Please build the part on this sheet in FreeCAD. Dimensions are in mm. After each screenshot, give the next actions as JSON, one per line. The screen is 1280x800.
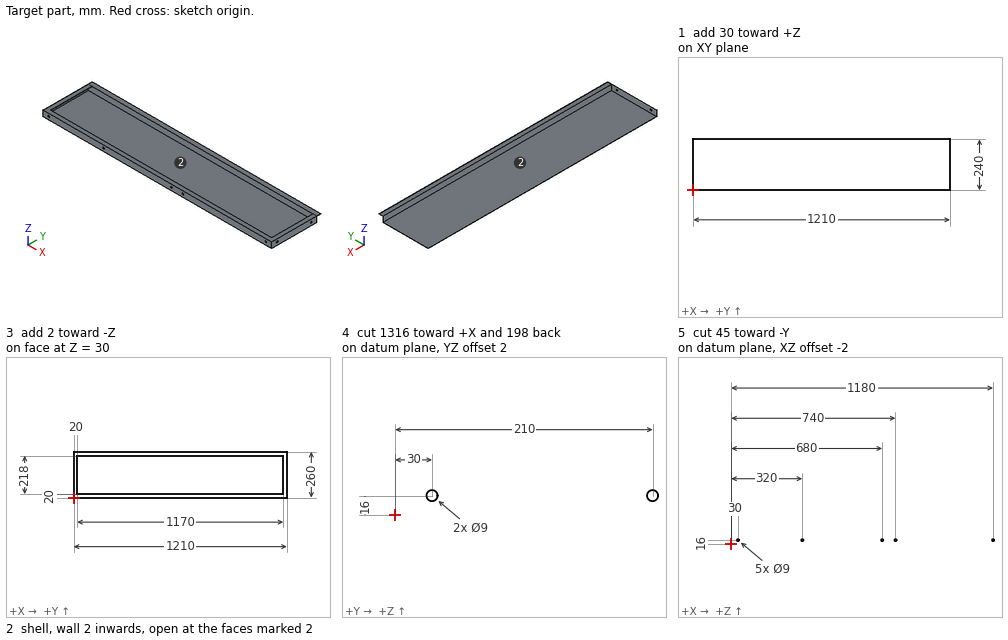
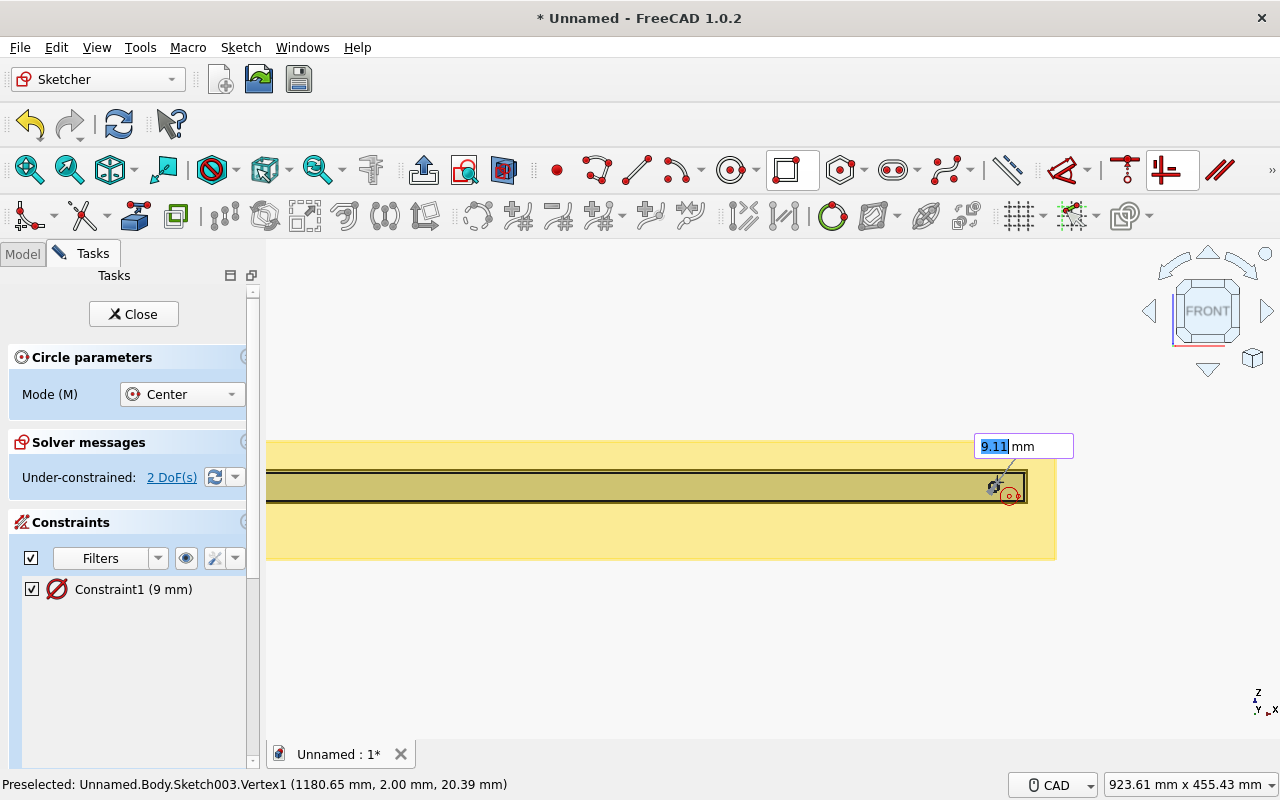
{"action": "type", "text": "9"}
{"action": "key", "text": "Return"}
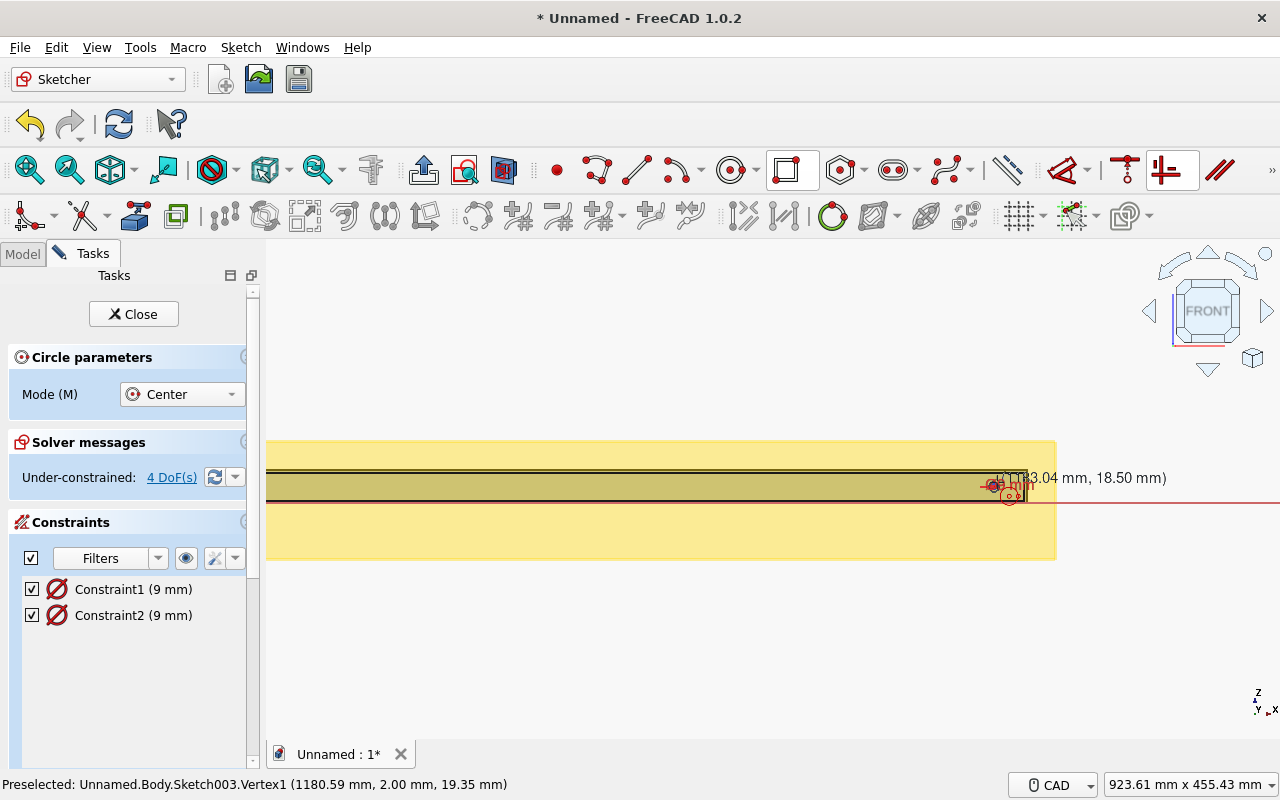
{"action": "scroll", "coordinate": [445, 486], "scroll_direction": "up", "scroll_amount": 8}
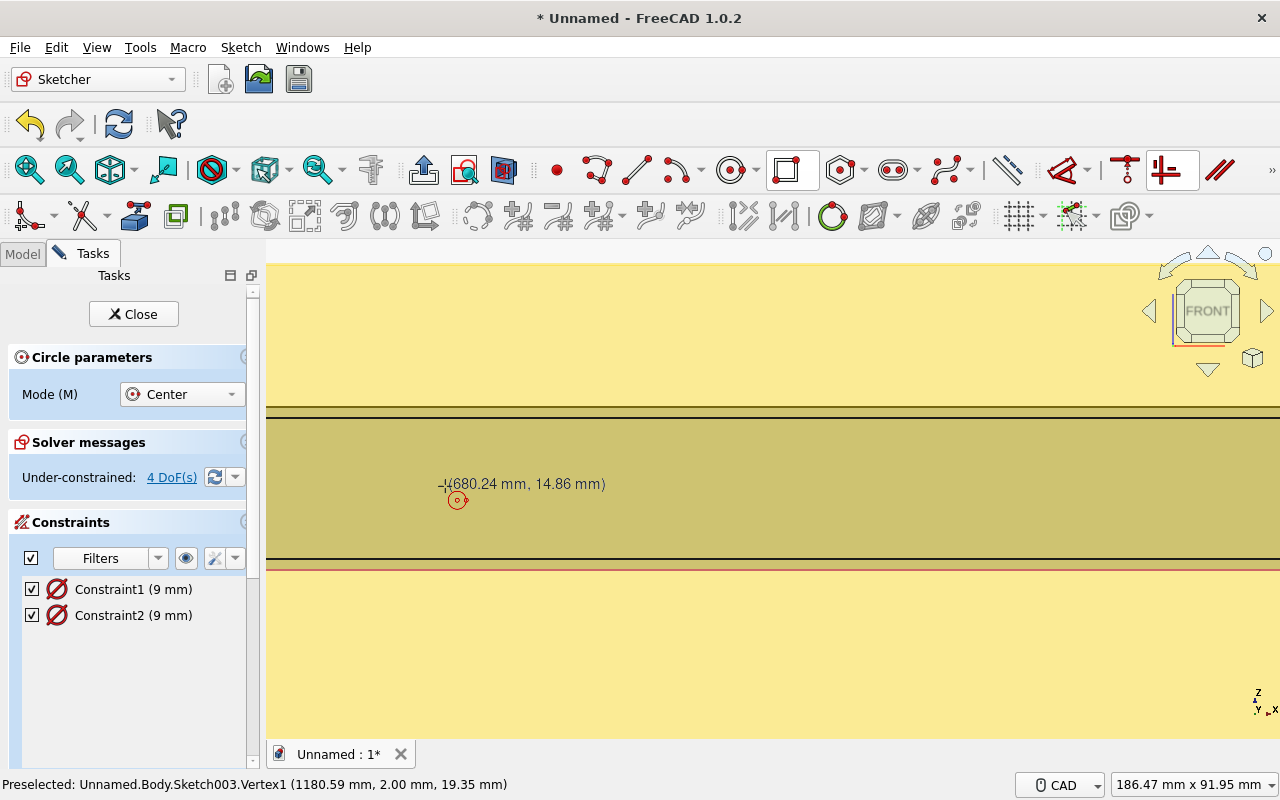
{"action": "scroll", "coordinate": [778, 486], "scroll_direction": "down", "scroll_amount": 12}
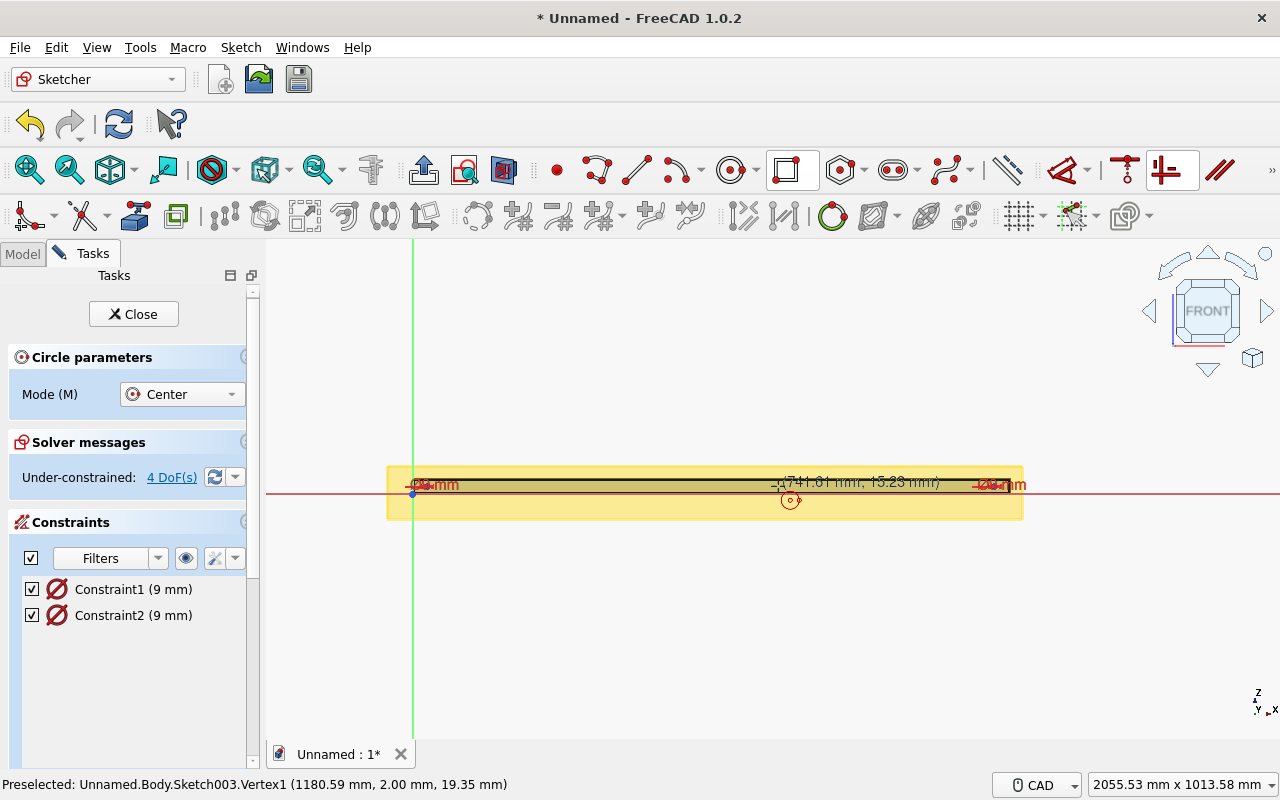
{"action": "scroll", "coordinate": [748, 486], "scroll_direction": "up", "scroll_amount": 4}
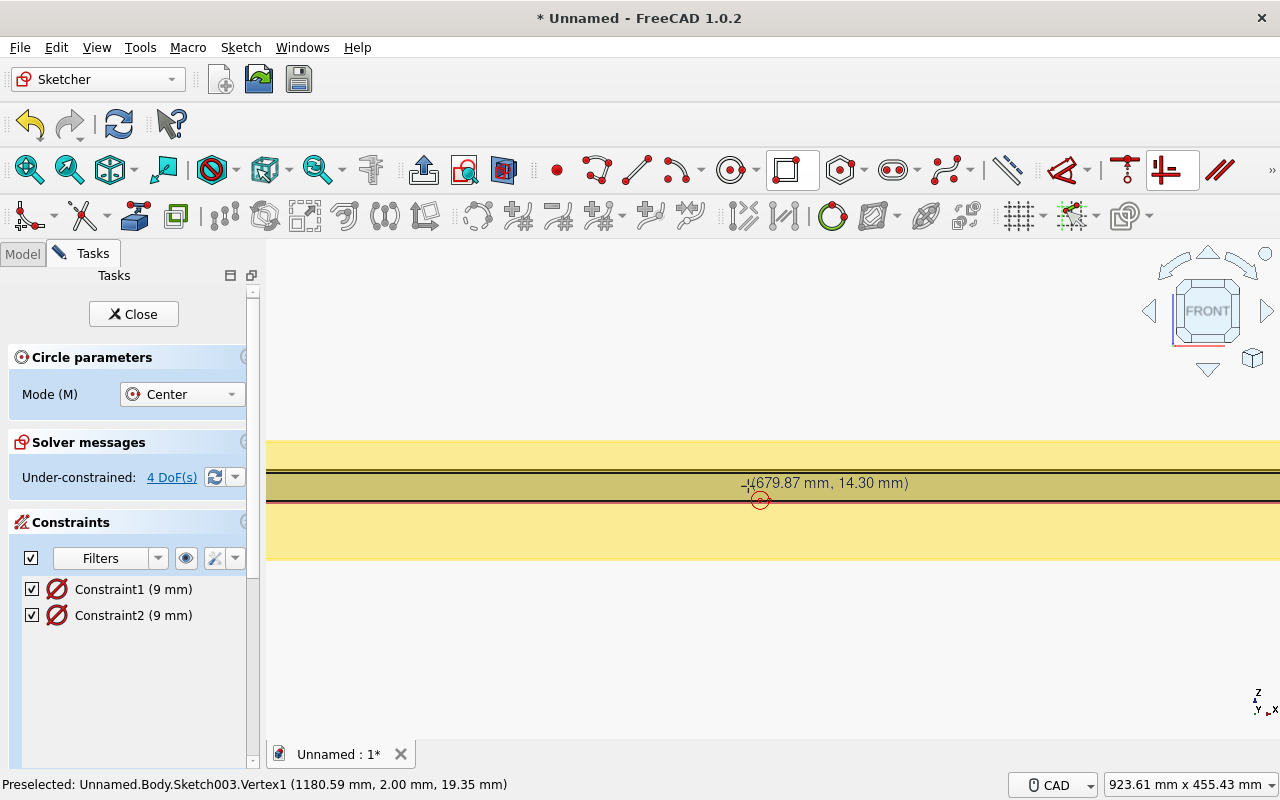
{"action": "left_click", "coordinate": [748, 486]}
{"action": "mouse_move", "coordinate": [751, 482]}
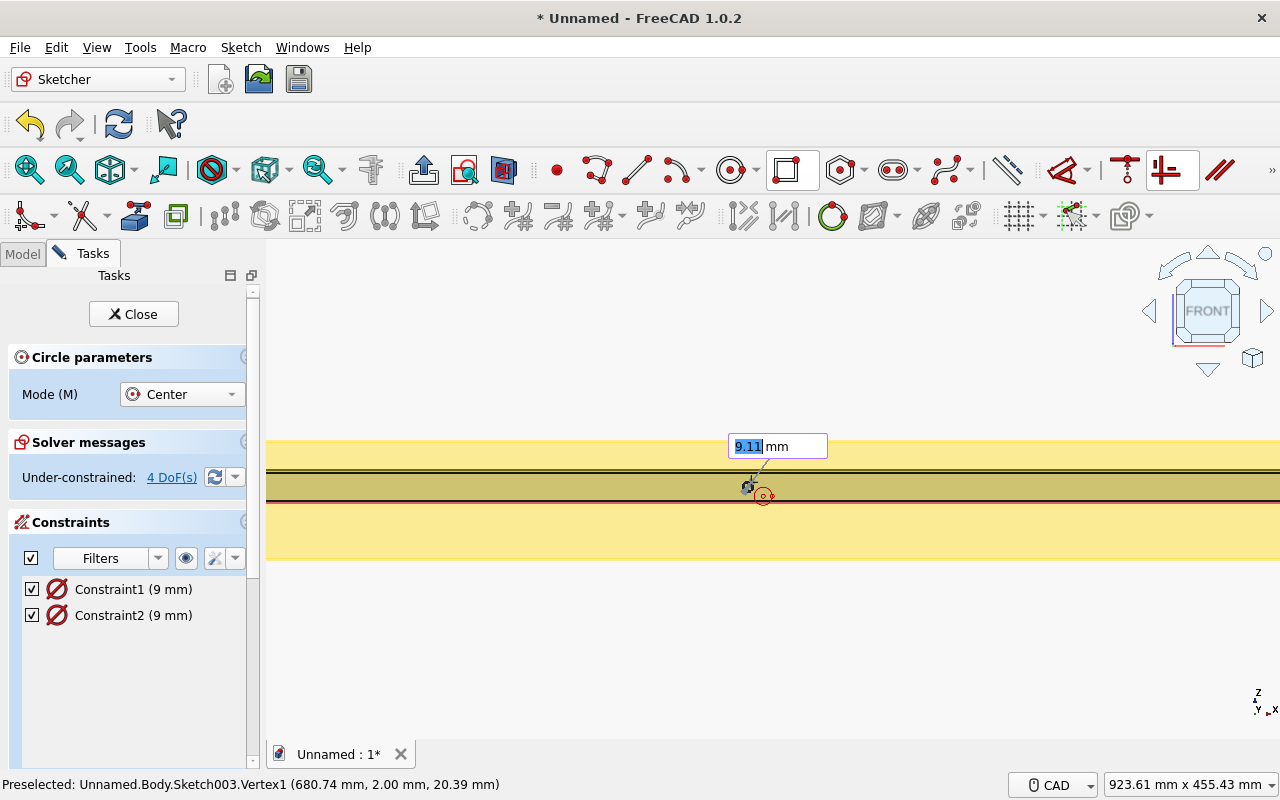
{"action": "type", "text": "9"}
{"action": "key", "text": "Return"}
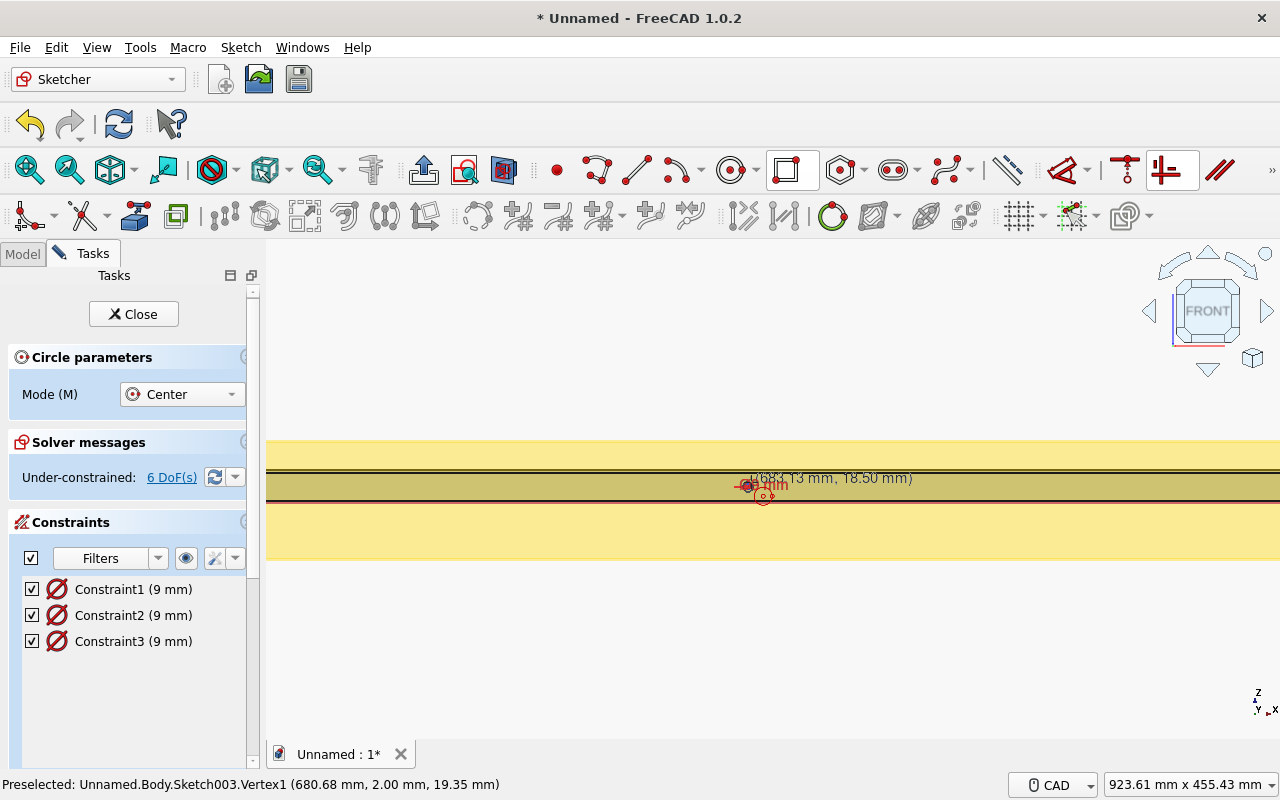
{"action": "scroll", "coordinate": [352, 486], "scroll_direction": "up", "scroll_amount": 8}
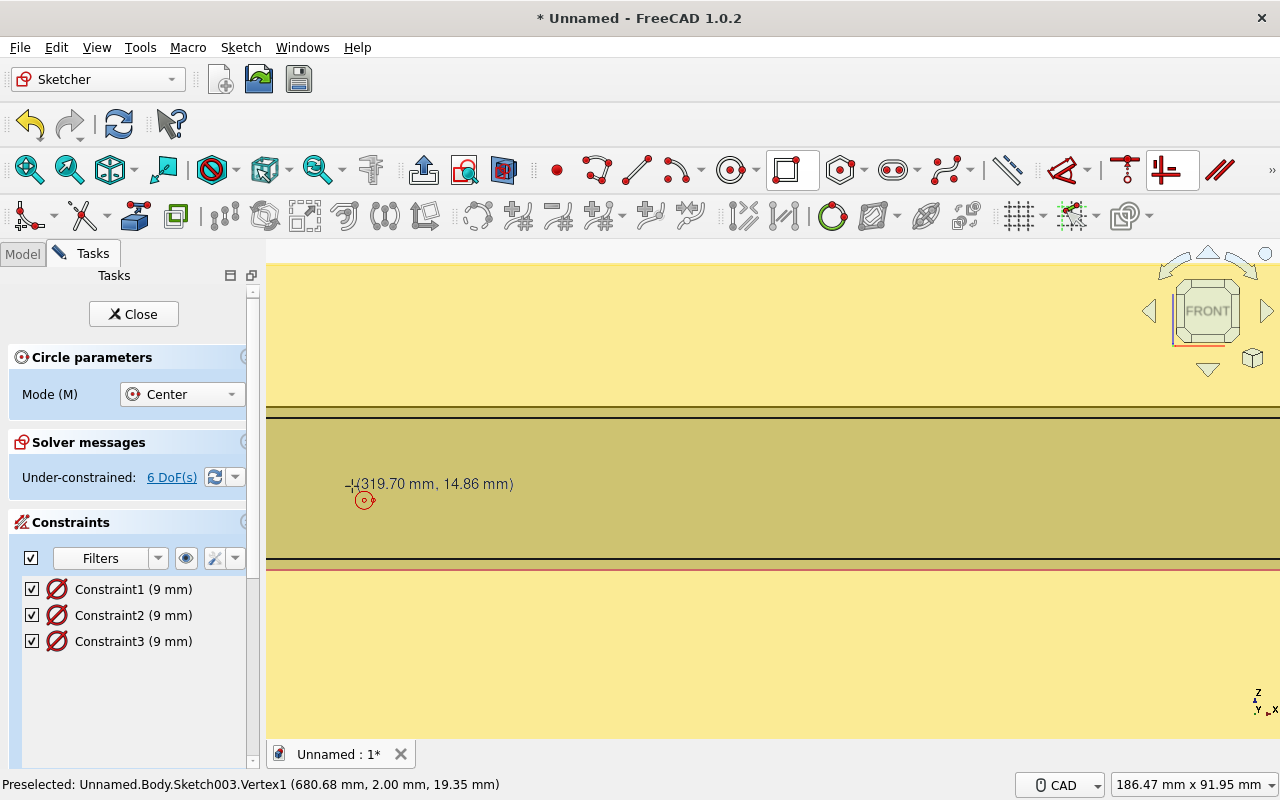
{"action": "scroll", "coordinate": [592, 486], "scroll_direction": "down", "scroll_amount": 12}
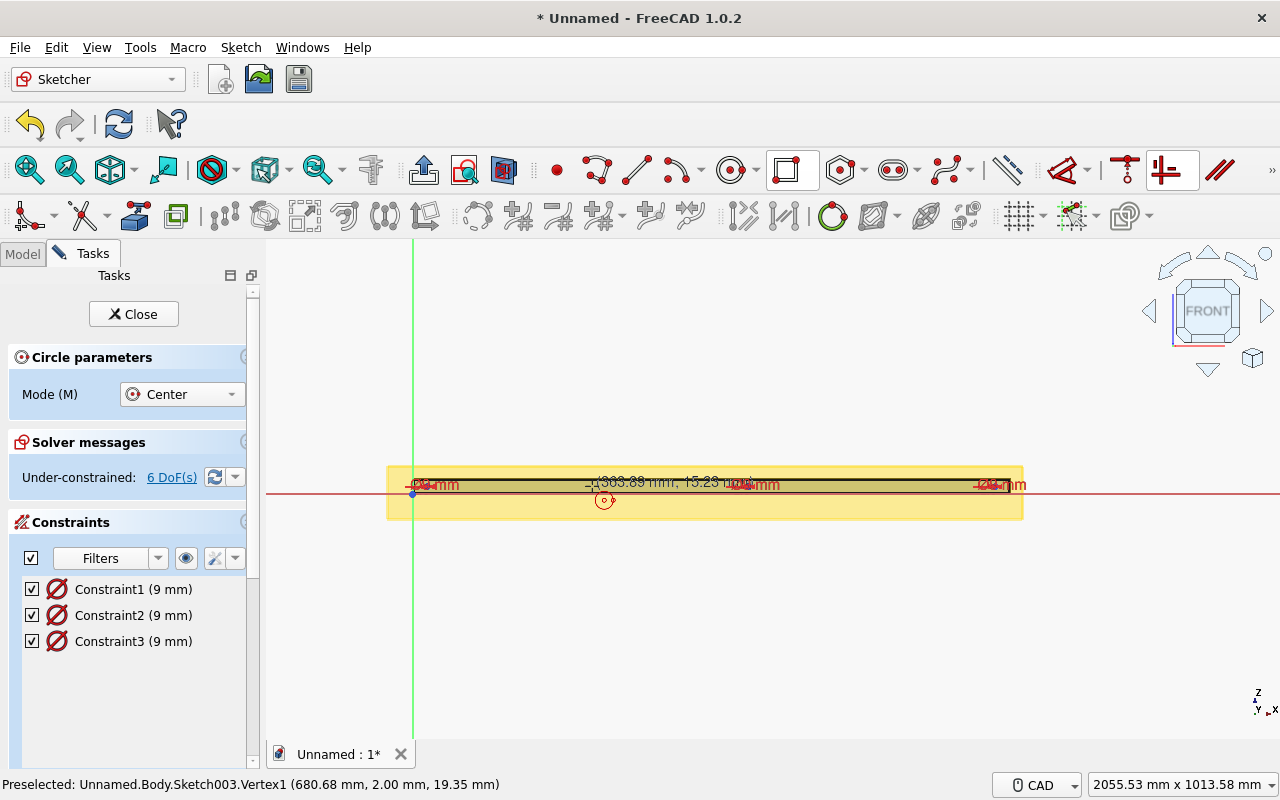
{"action": "scroll", "coordinate": [571, 486], "scroll_direction": "up", "scroll_amount": 4}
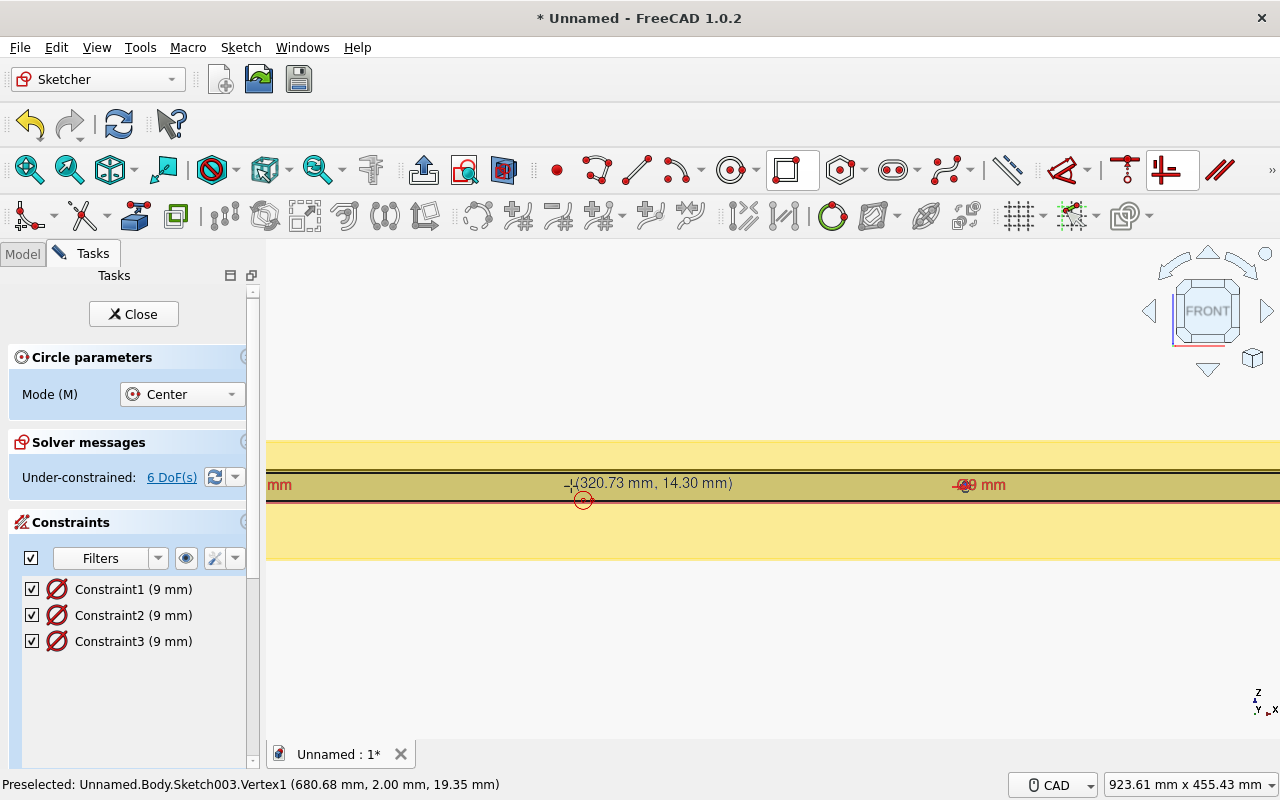
{"action": "left_click", "coordinate": [570, 486]}
{"action": "mouse_move", "coordinate": [573, 482]}